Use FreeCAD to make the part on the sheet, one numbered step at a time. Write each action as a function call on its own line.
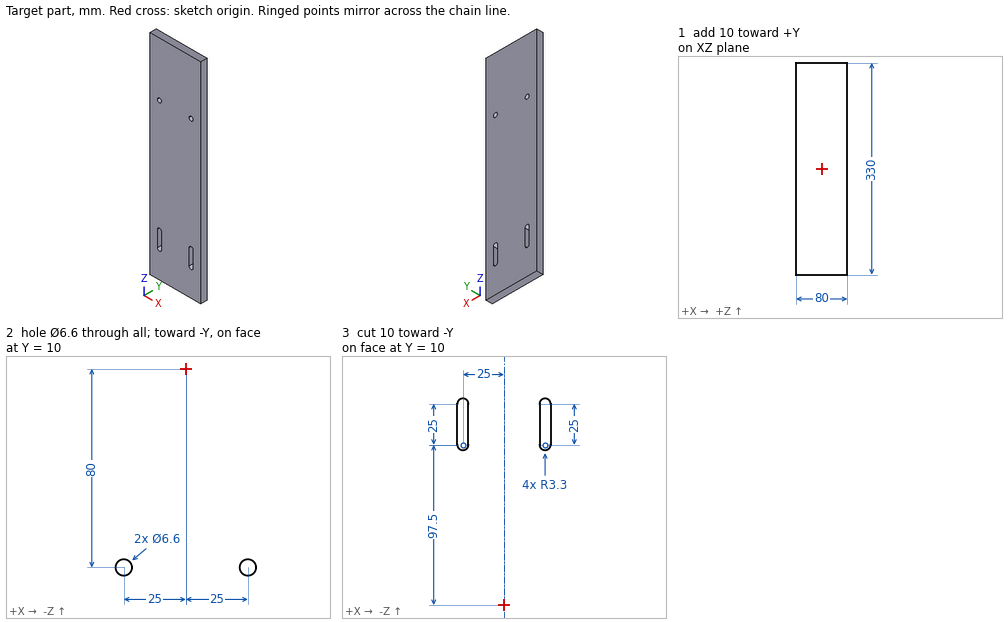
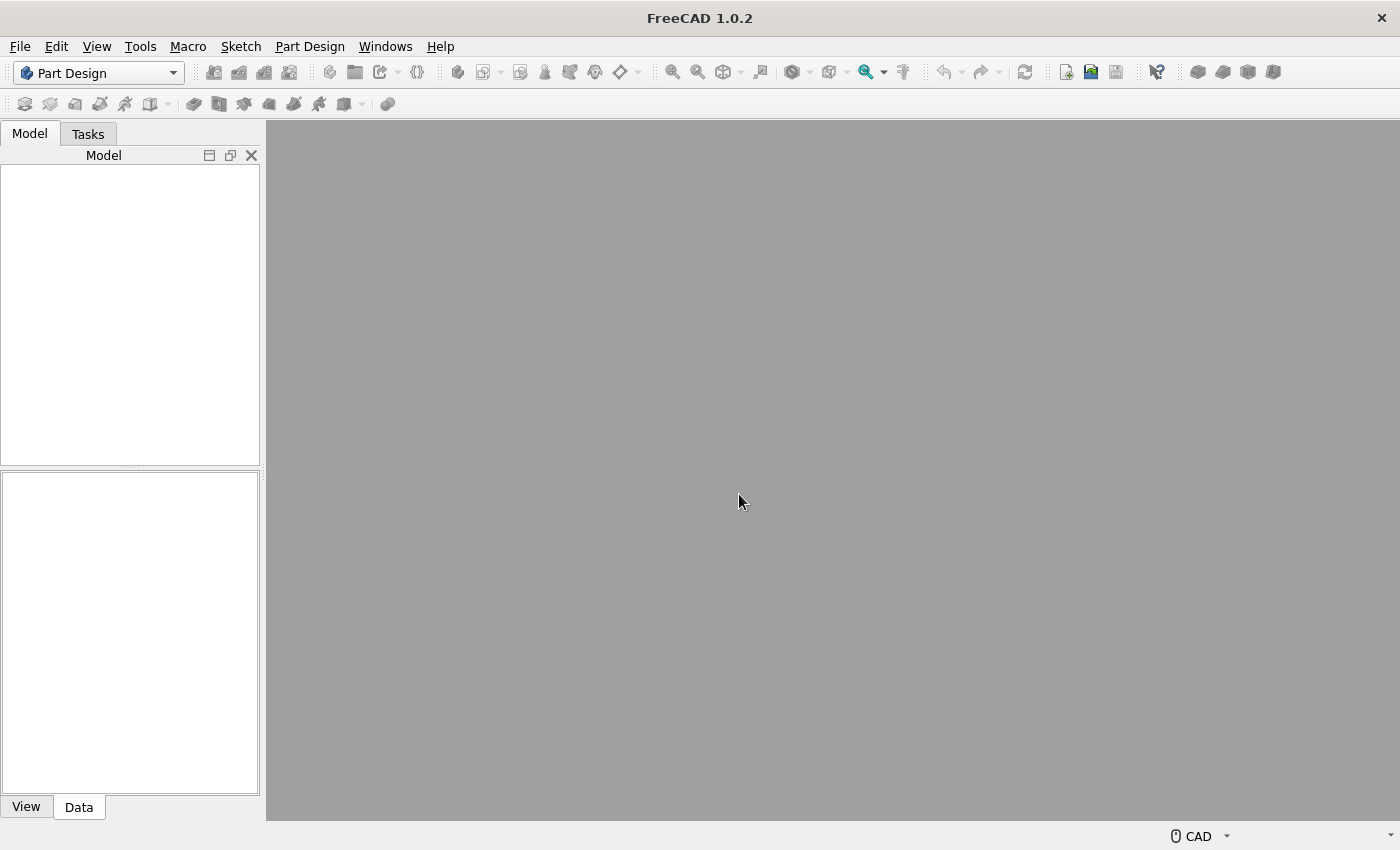
key(ctrl+n)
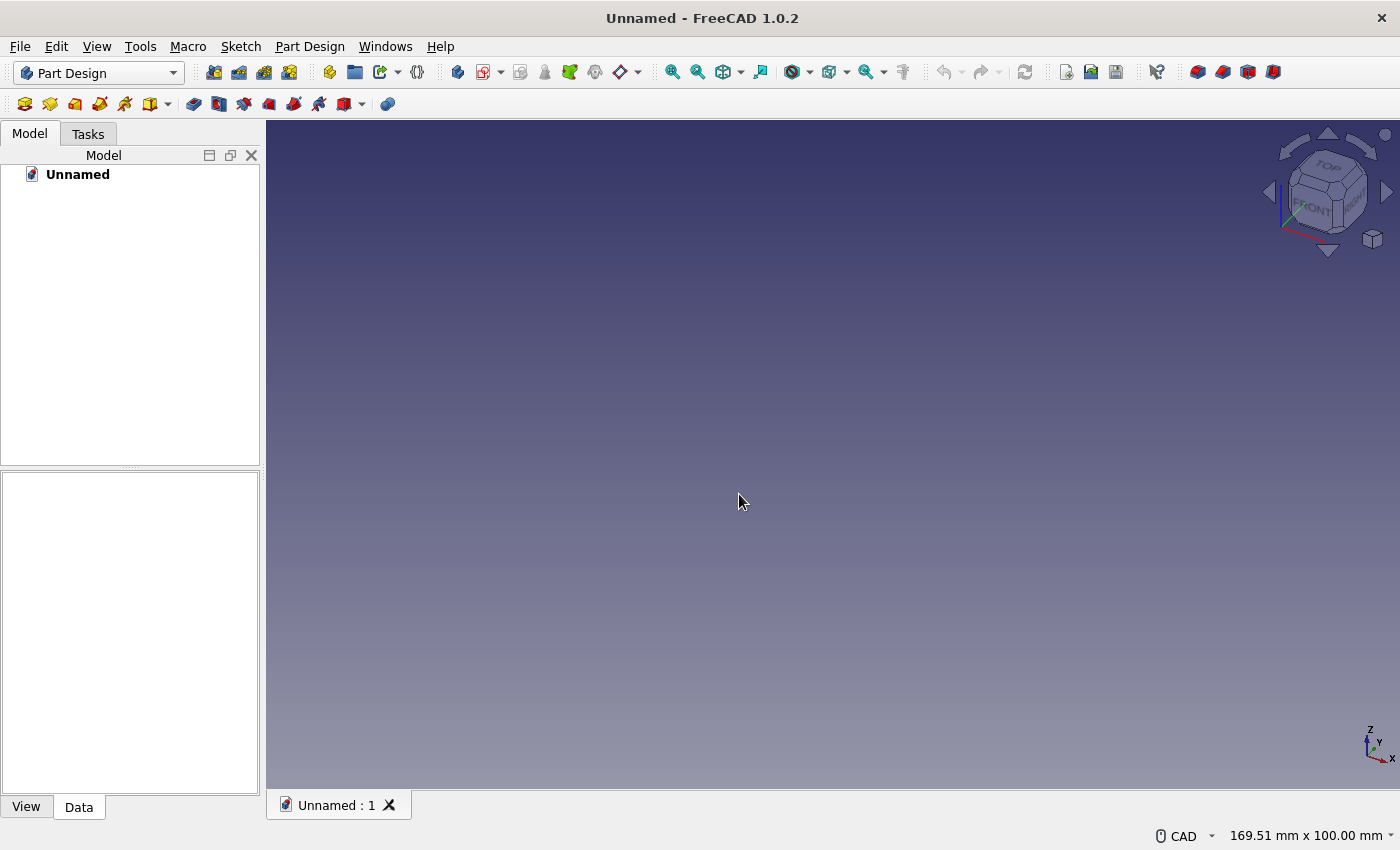
click(482, 72)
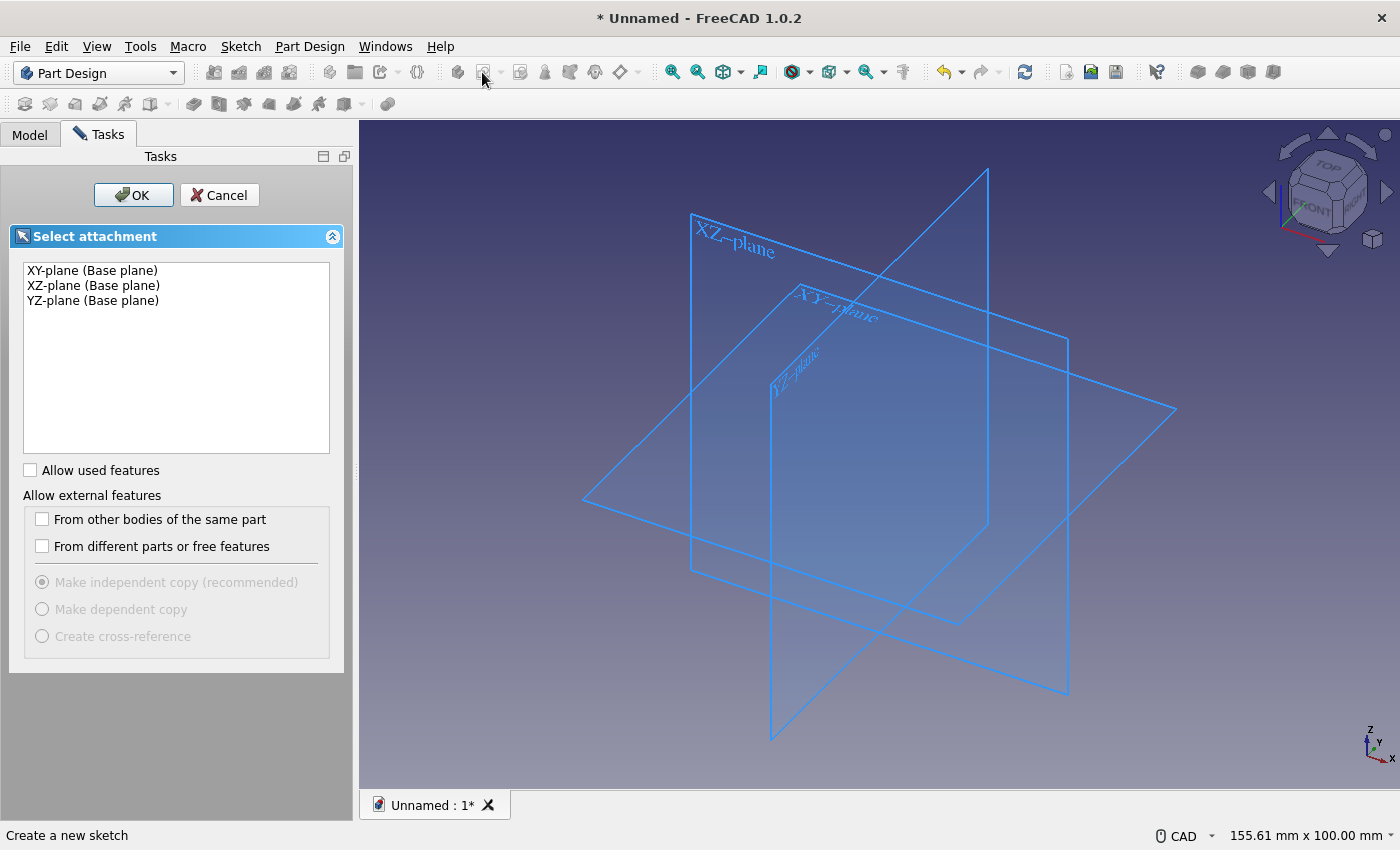
click(84, 286)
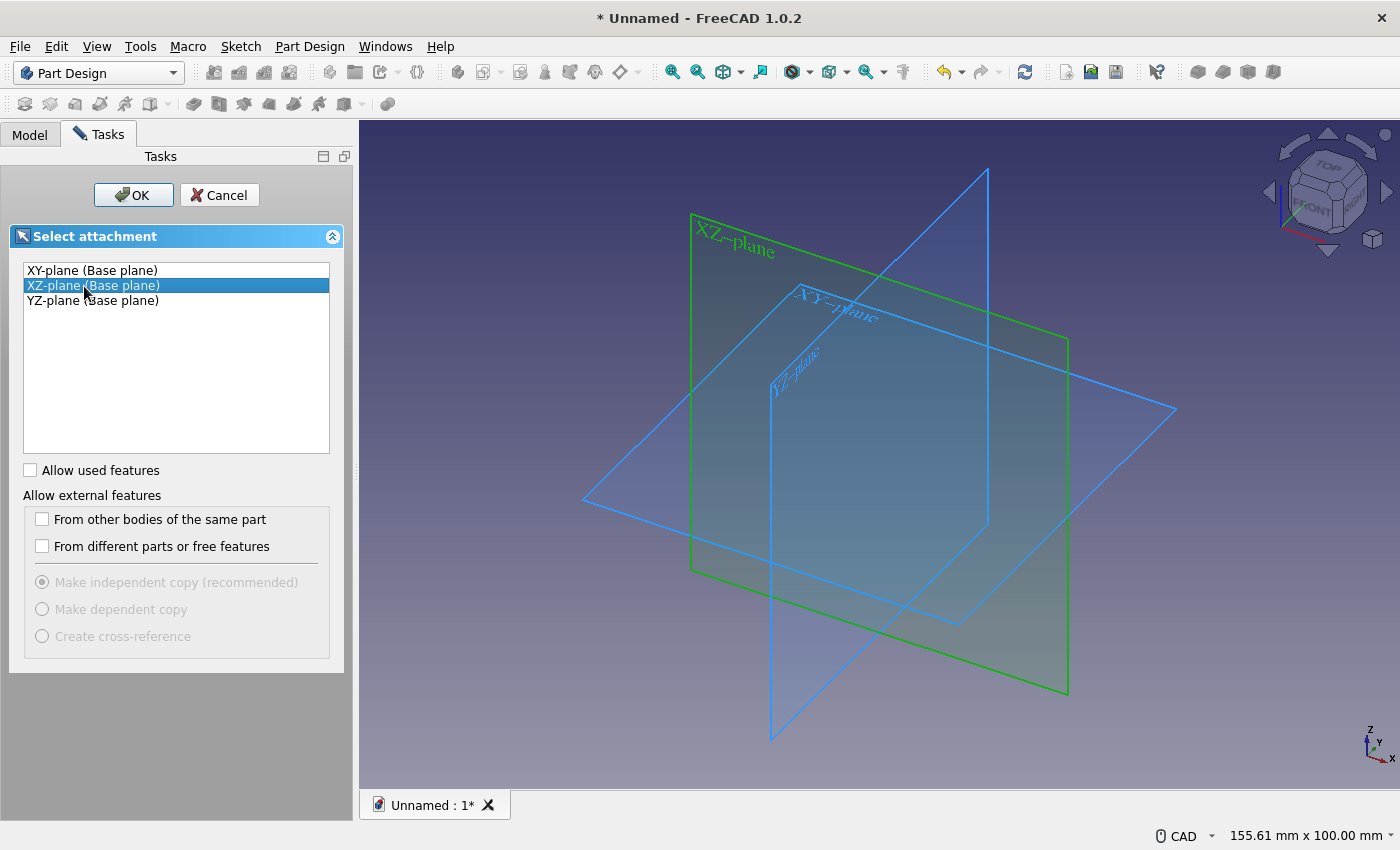
click(134, 195)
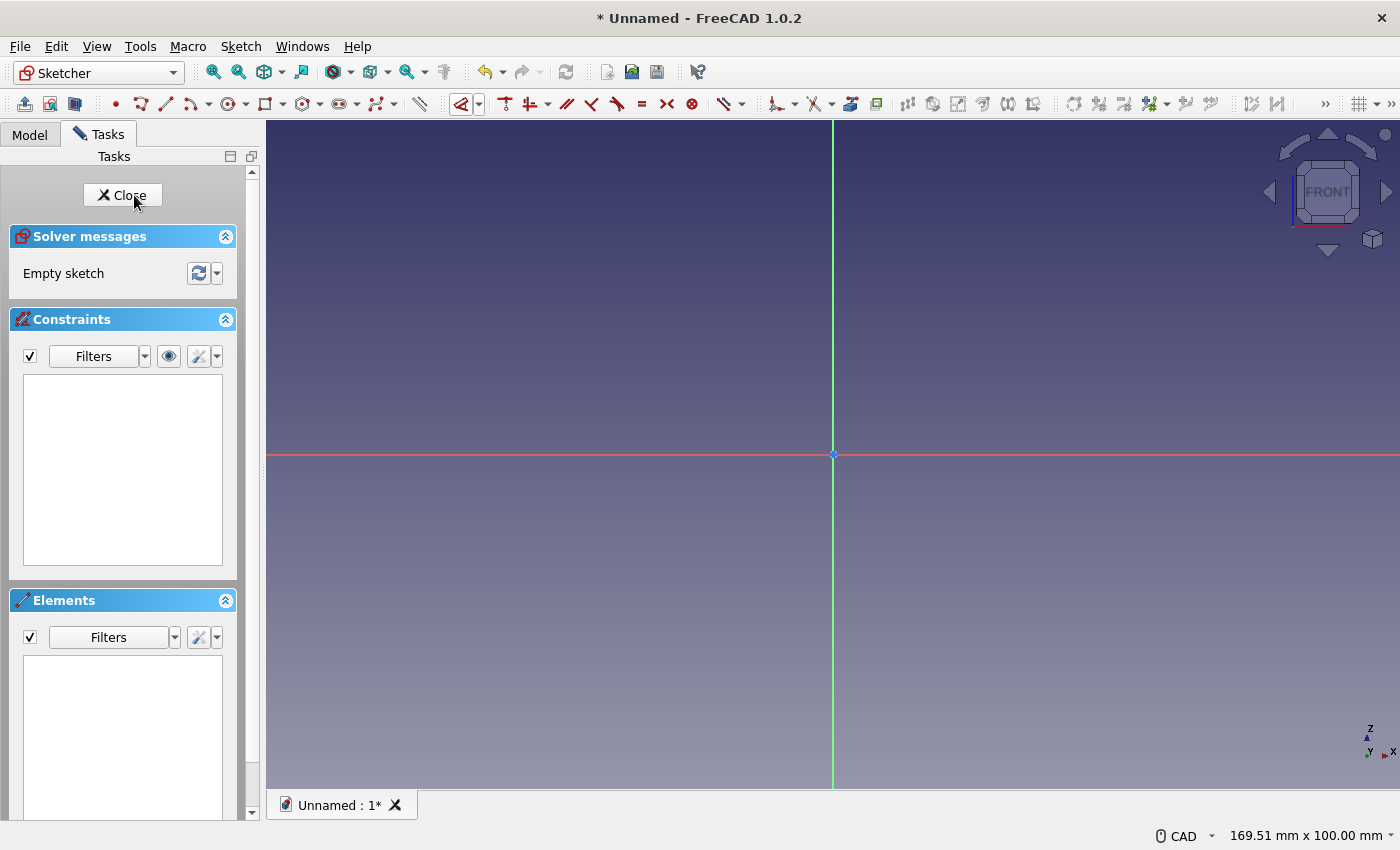
scroll(747, 454, down, 8)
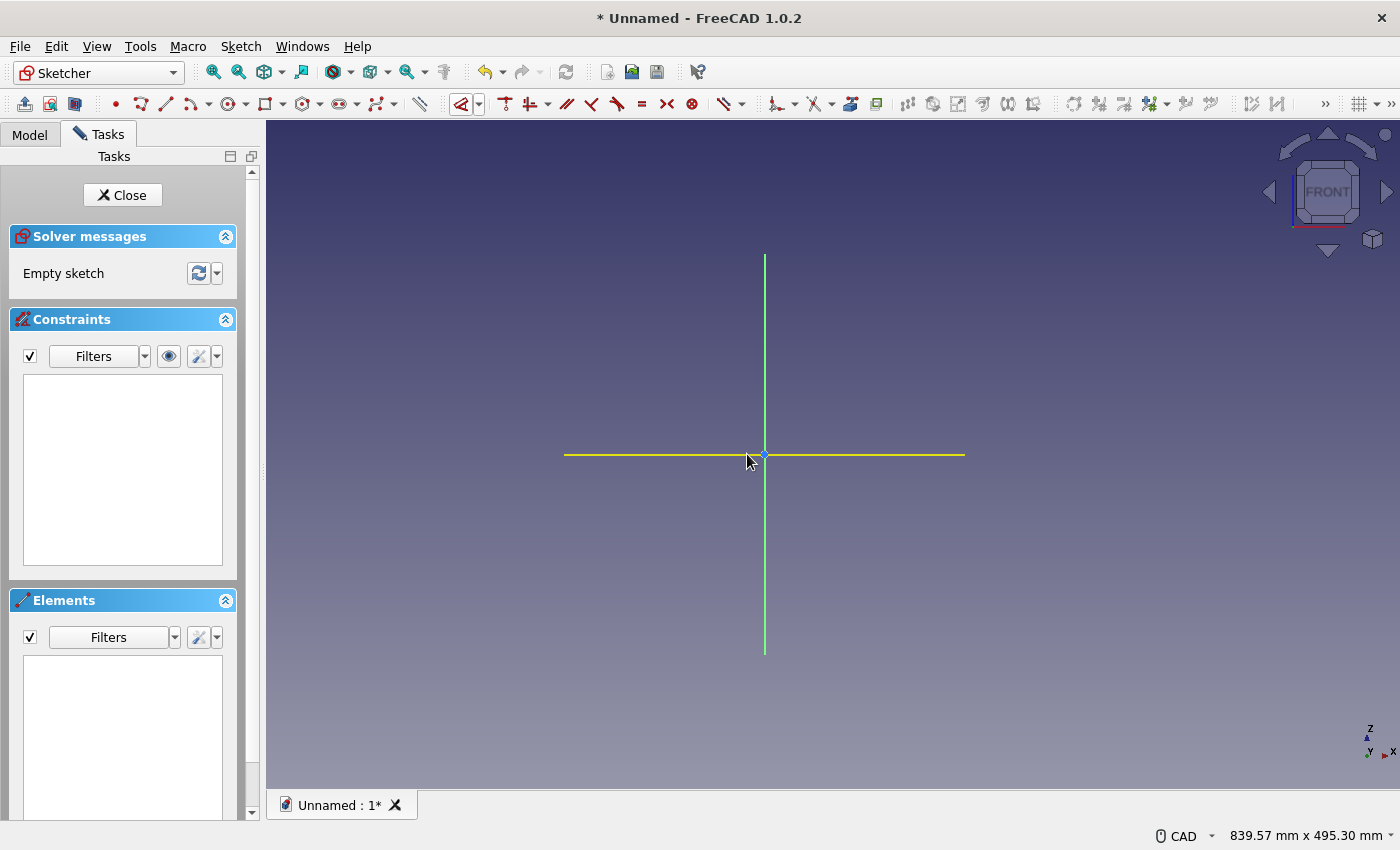
key(g)
key(v)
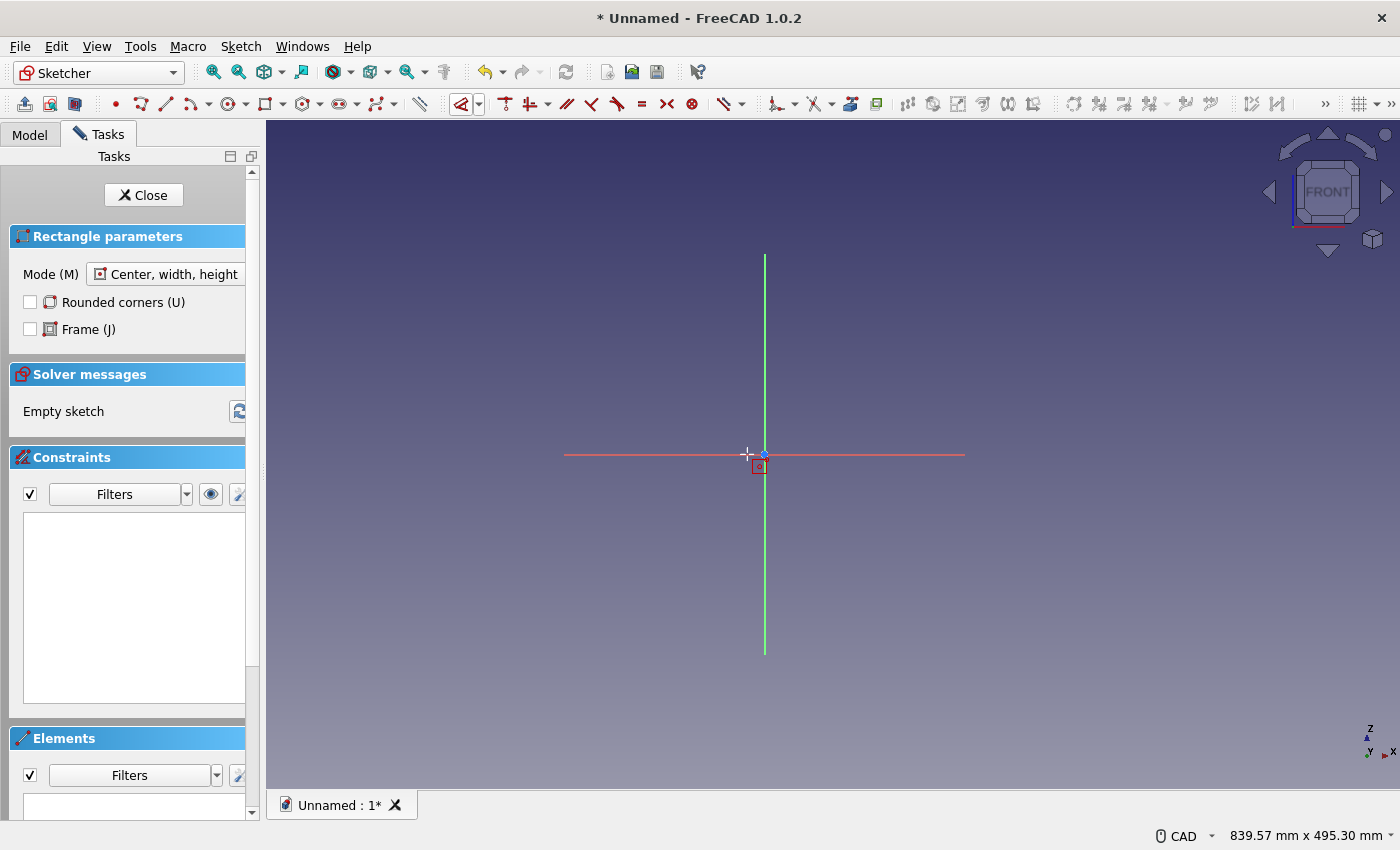
click(765, 454)
move(819, 232)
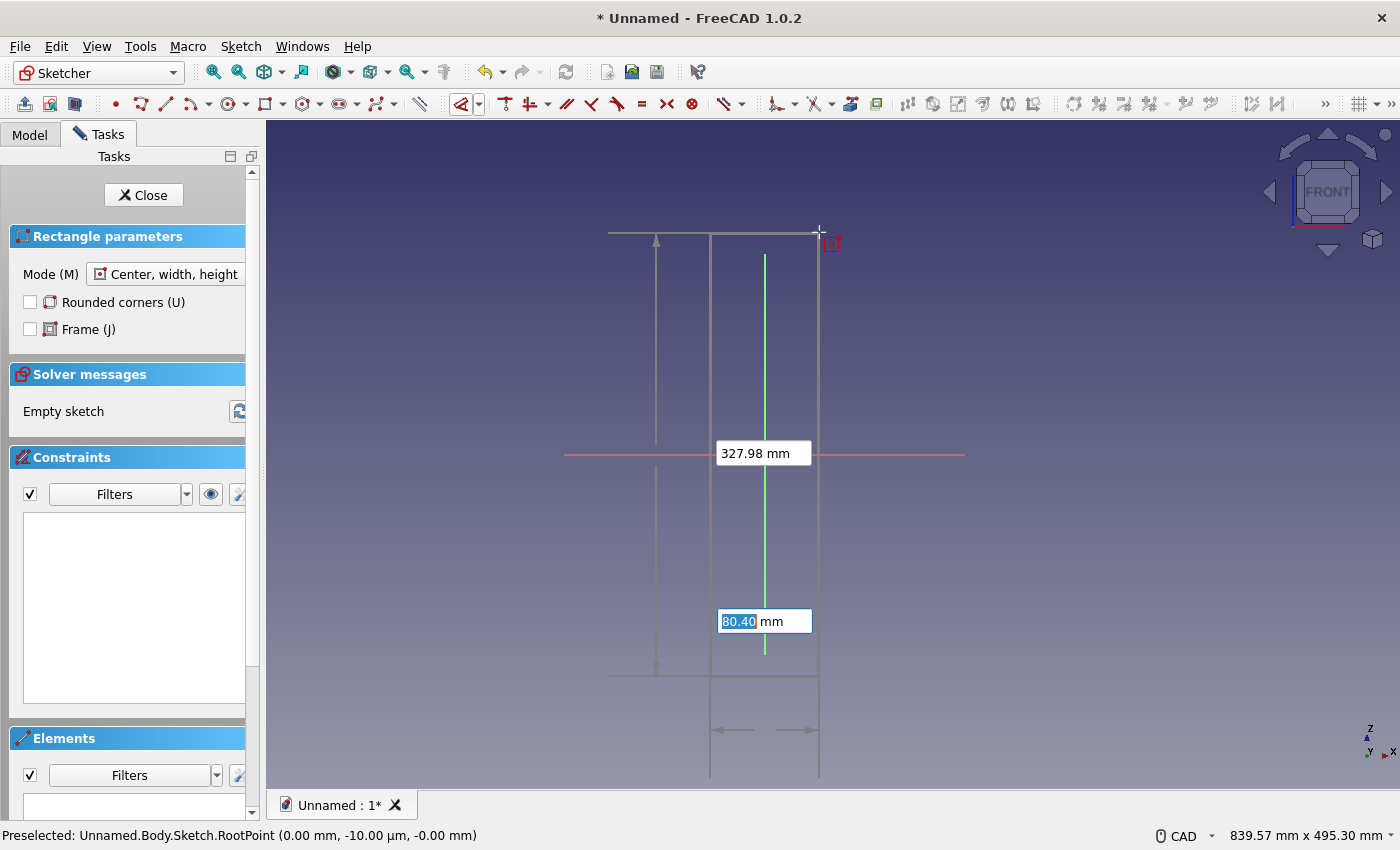
text(80)
key(Tab)
text(330)
key(Return)
key(Escape)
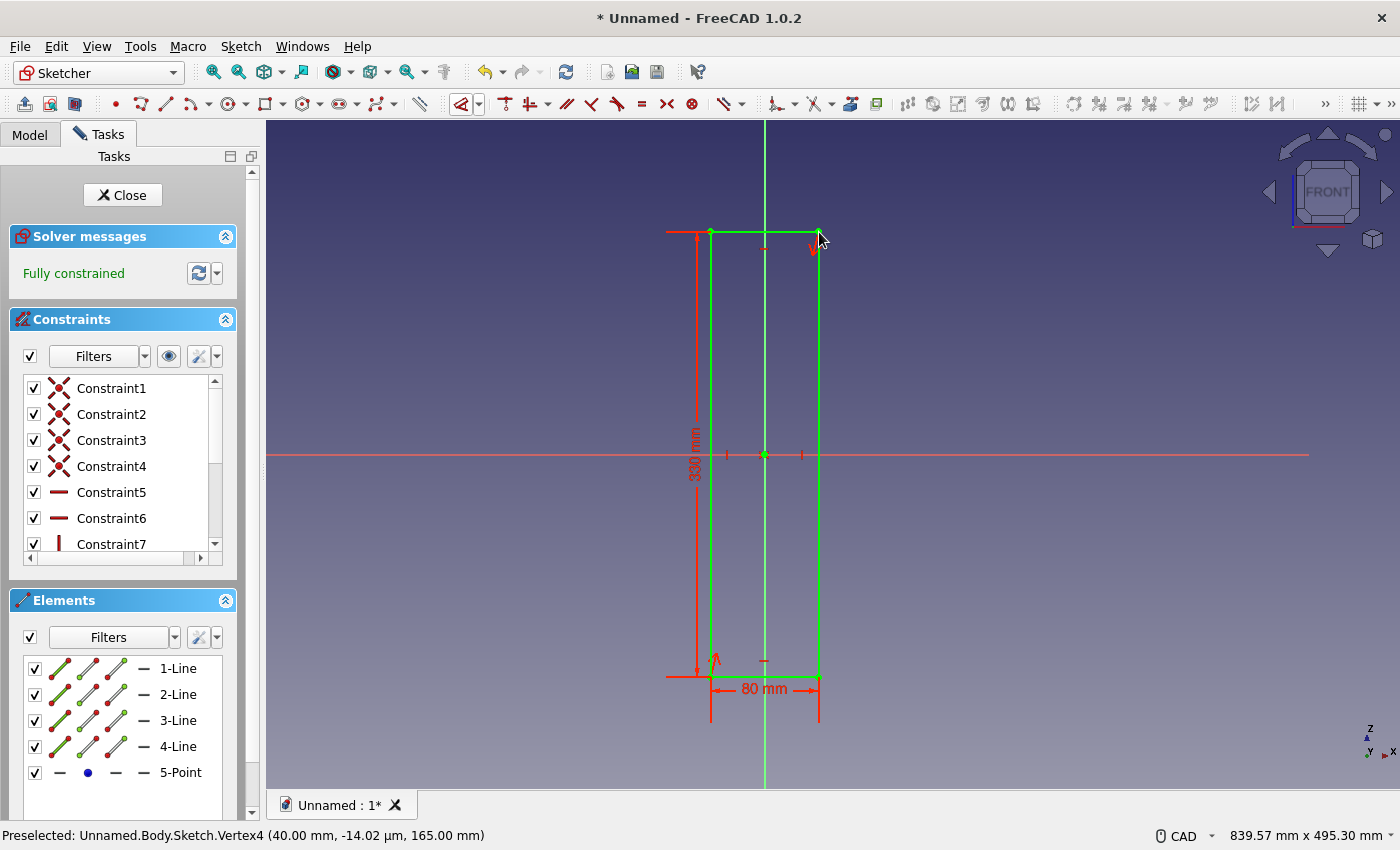
click(123, 195)